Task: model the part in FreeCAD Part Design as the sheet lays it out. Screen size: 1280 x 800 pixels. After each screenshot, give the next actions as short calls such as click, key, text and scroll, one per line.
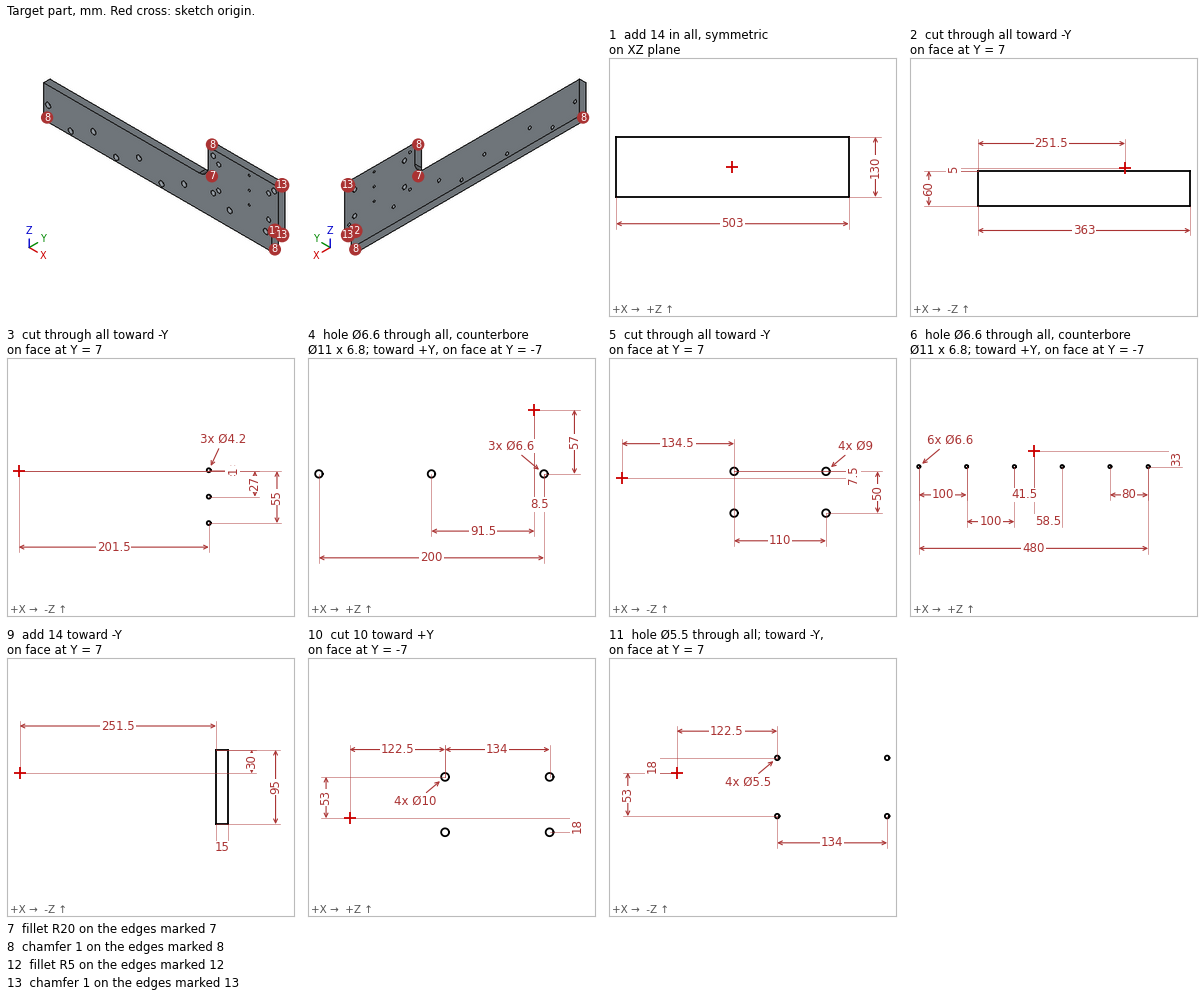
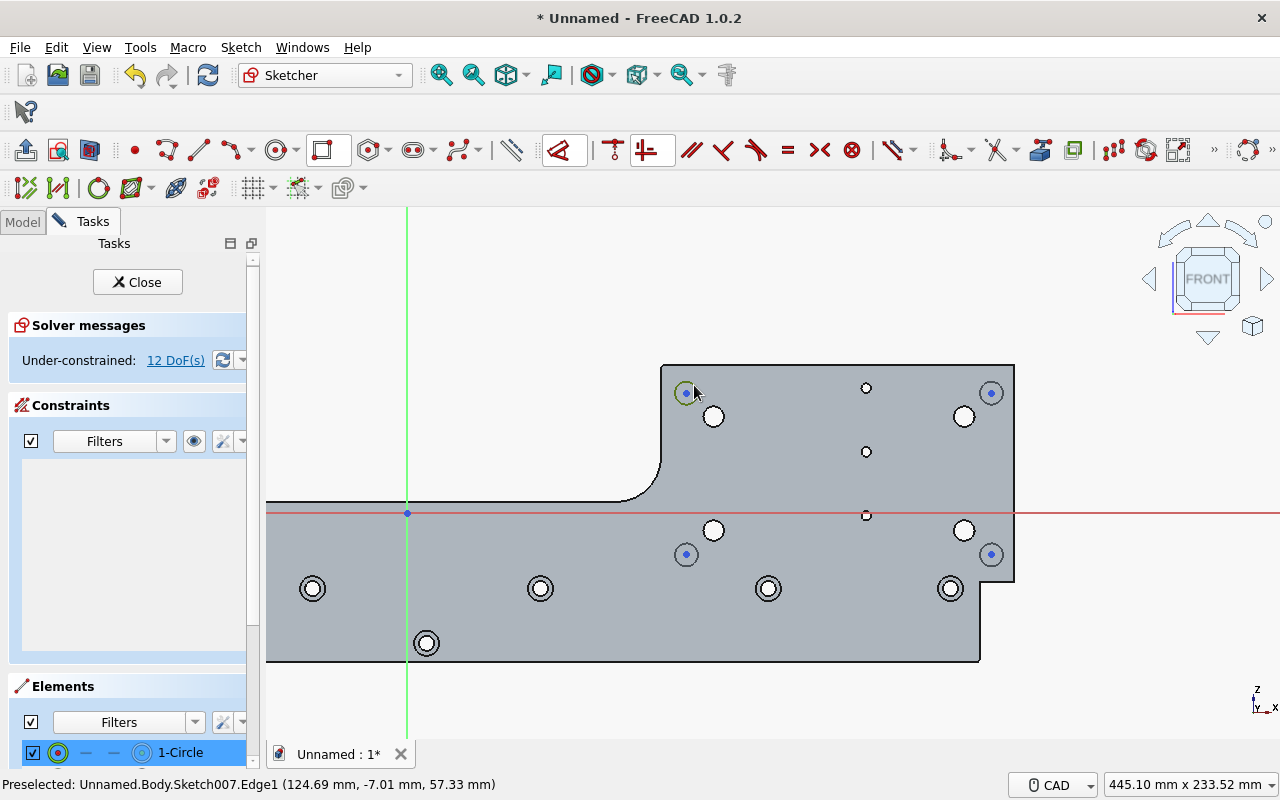
click(1000, 385)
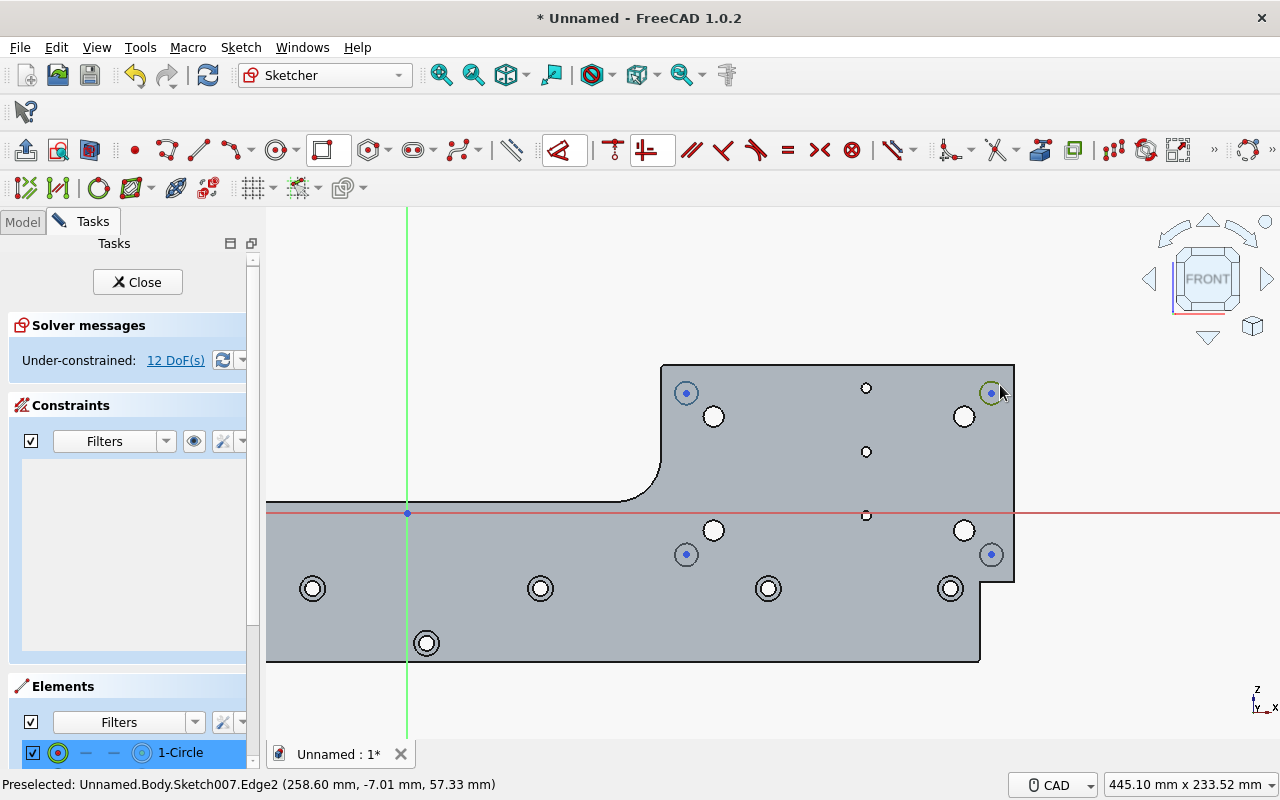
click(1000, 547)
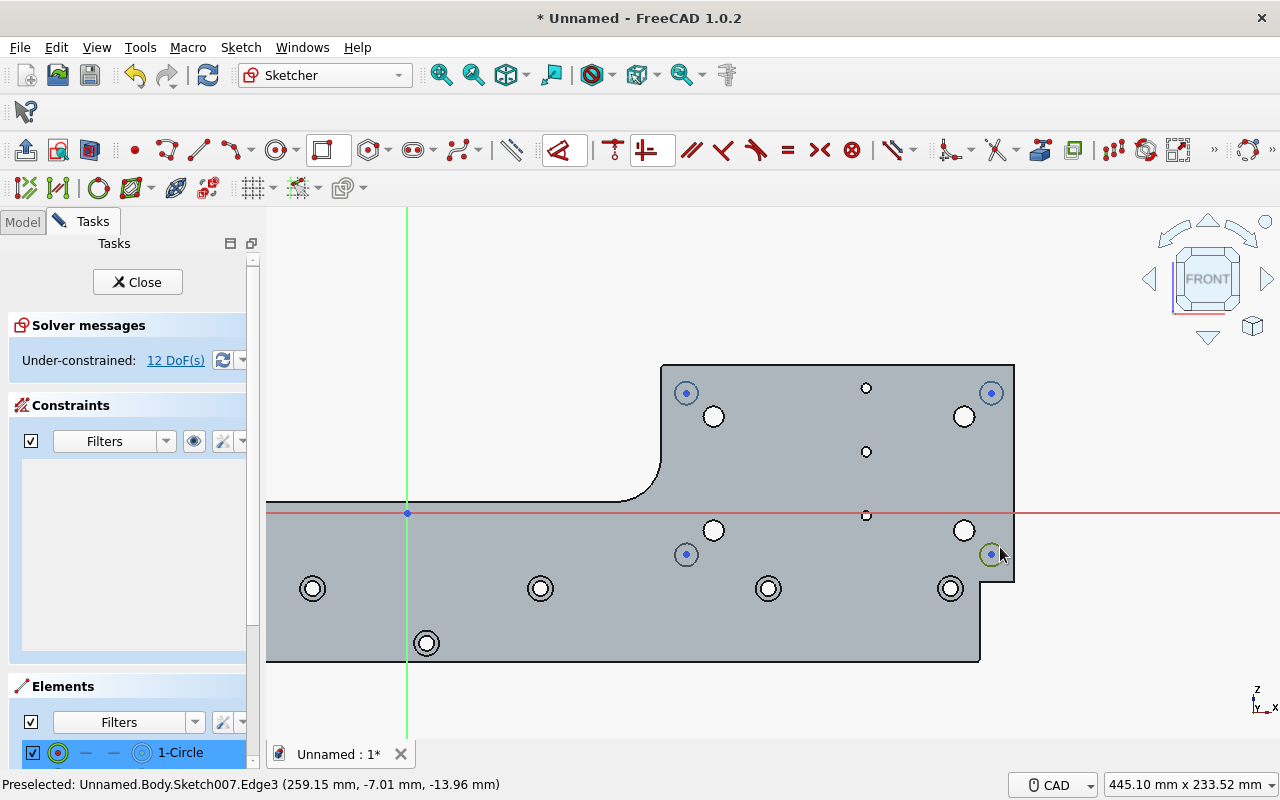
click(694, 547)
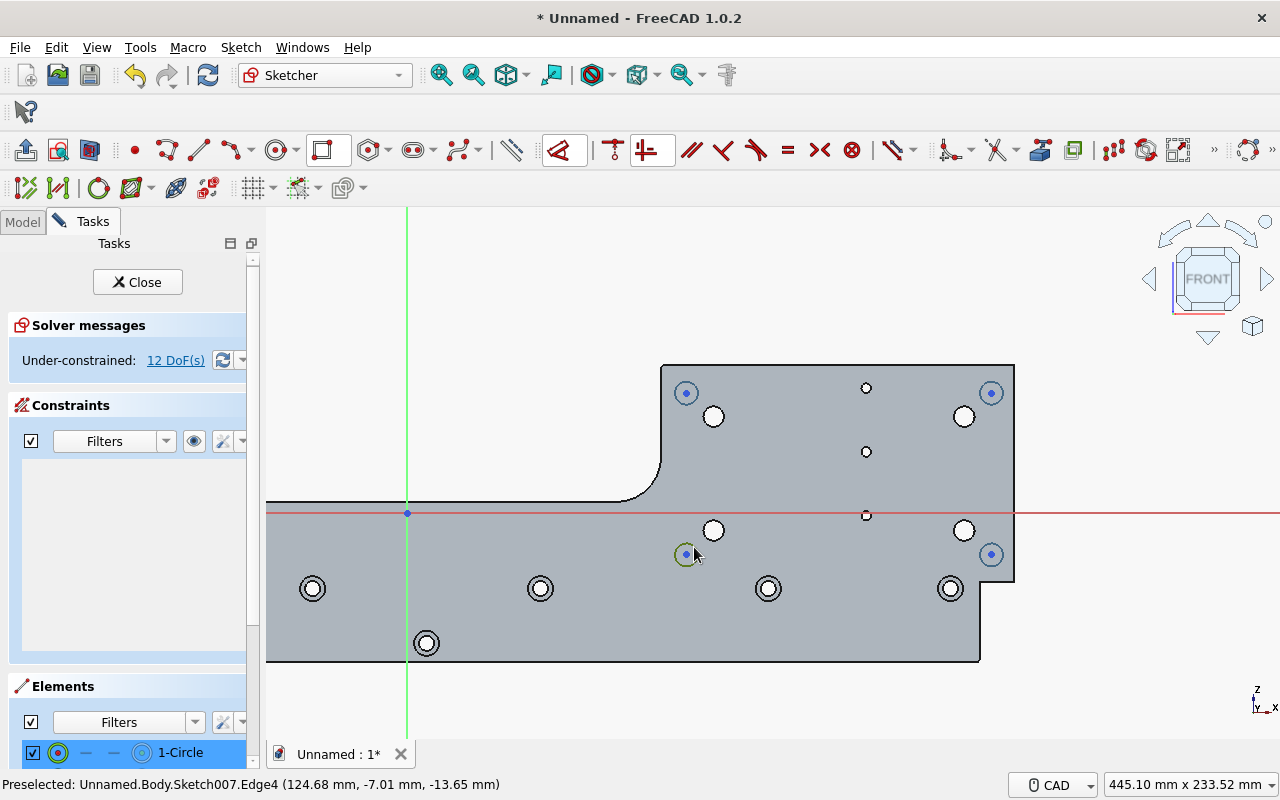
click(788, 150)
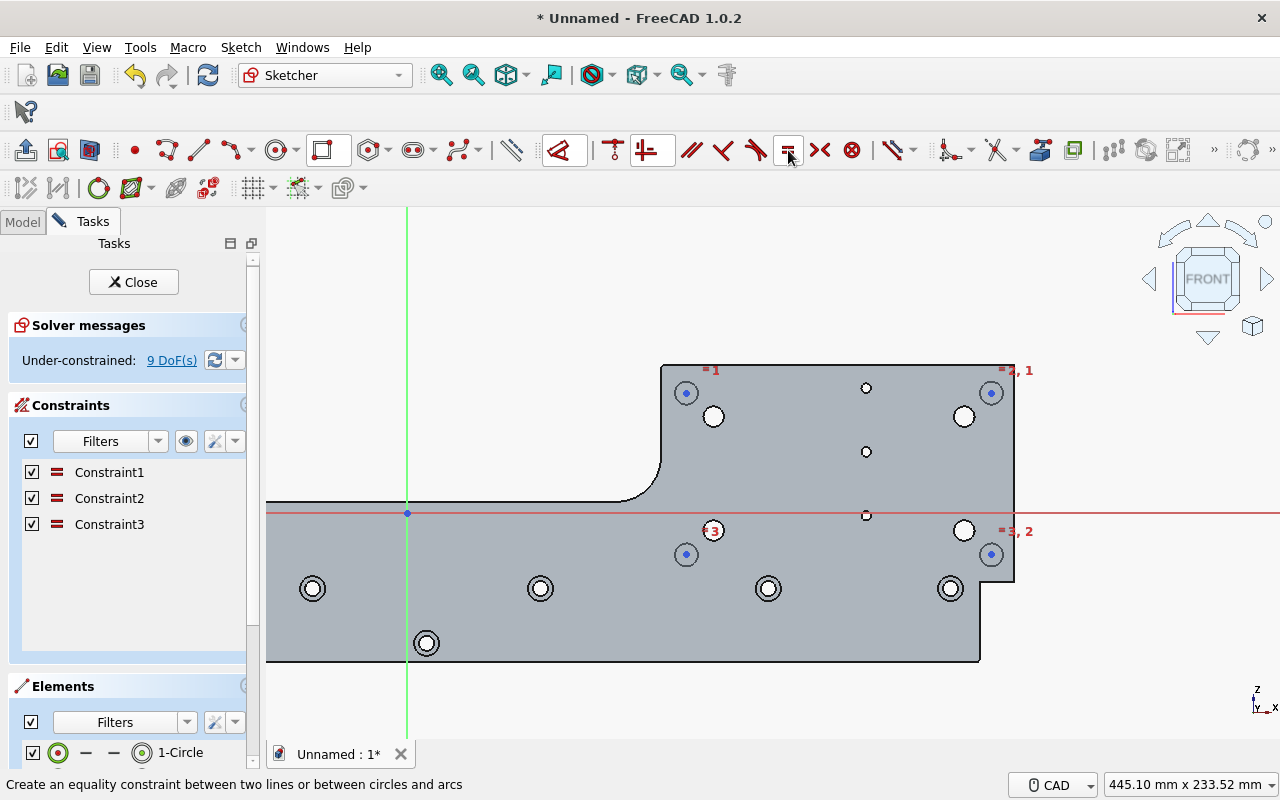
click(686, 393)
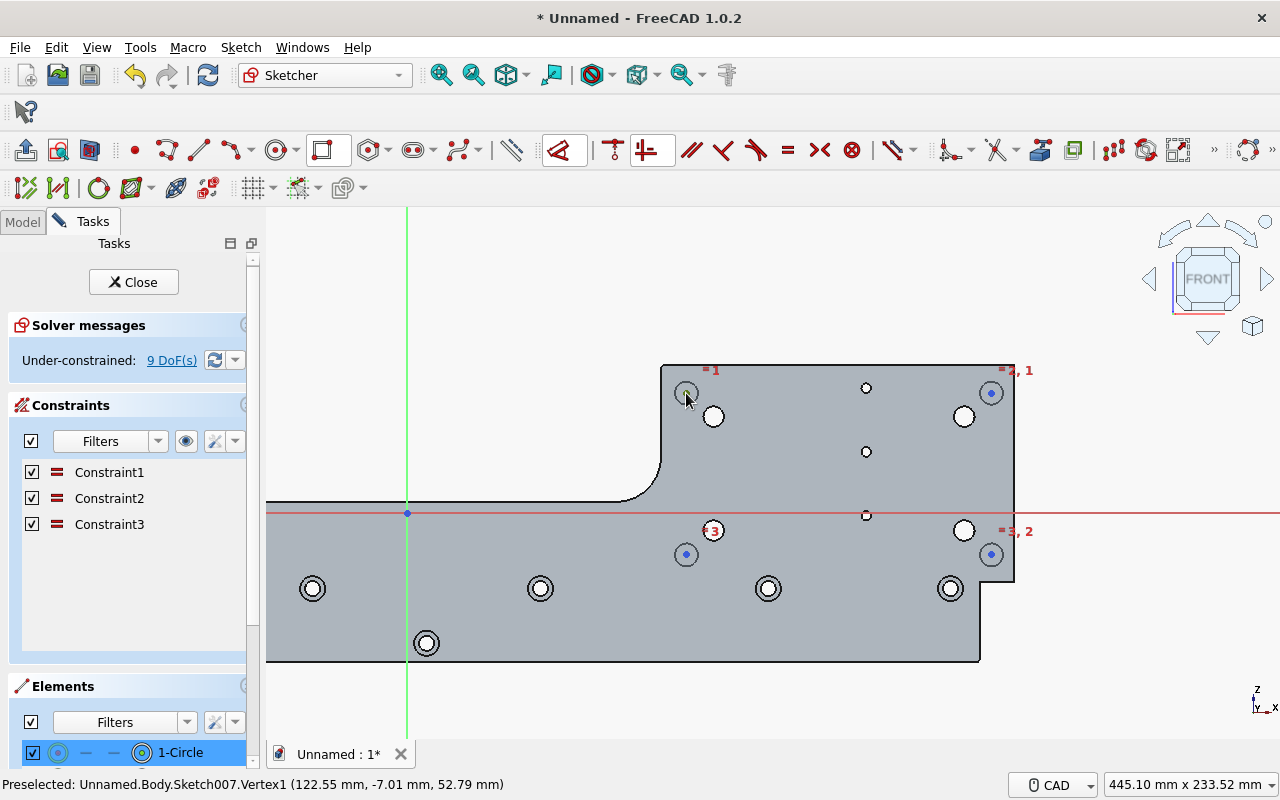
click(991, 393)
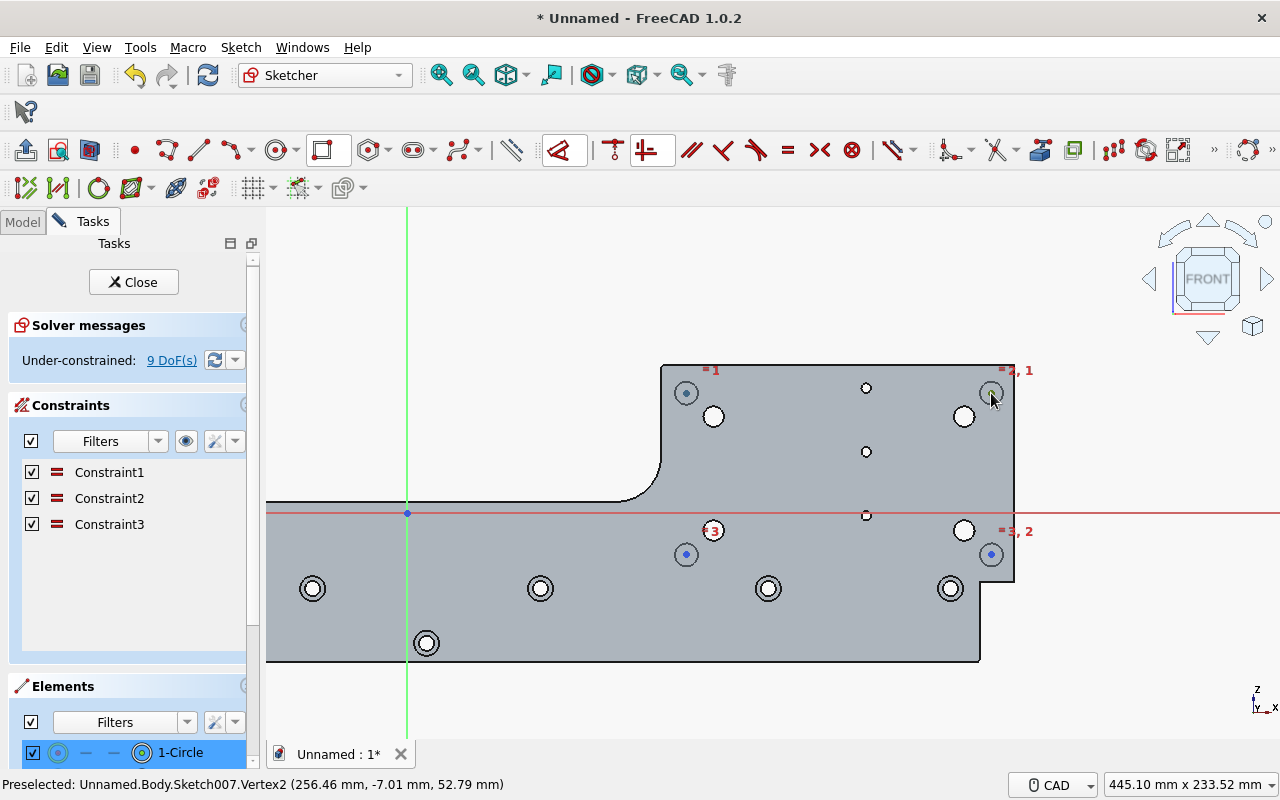
key(h)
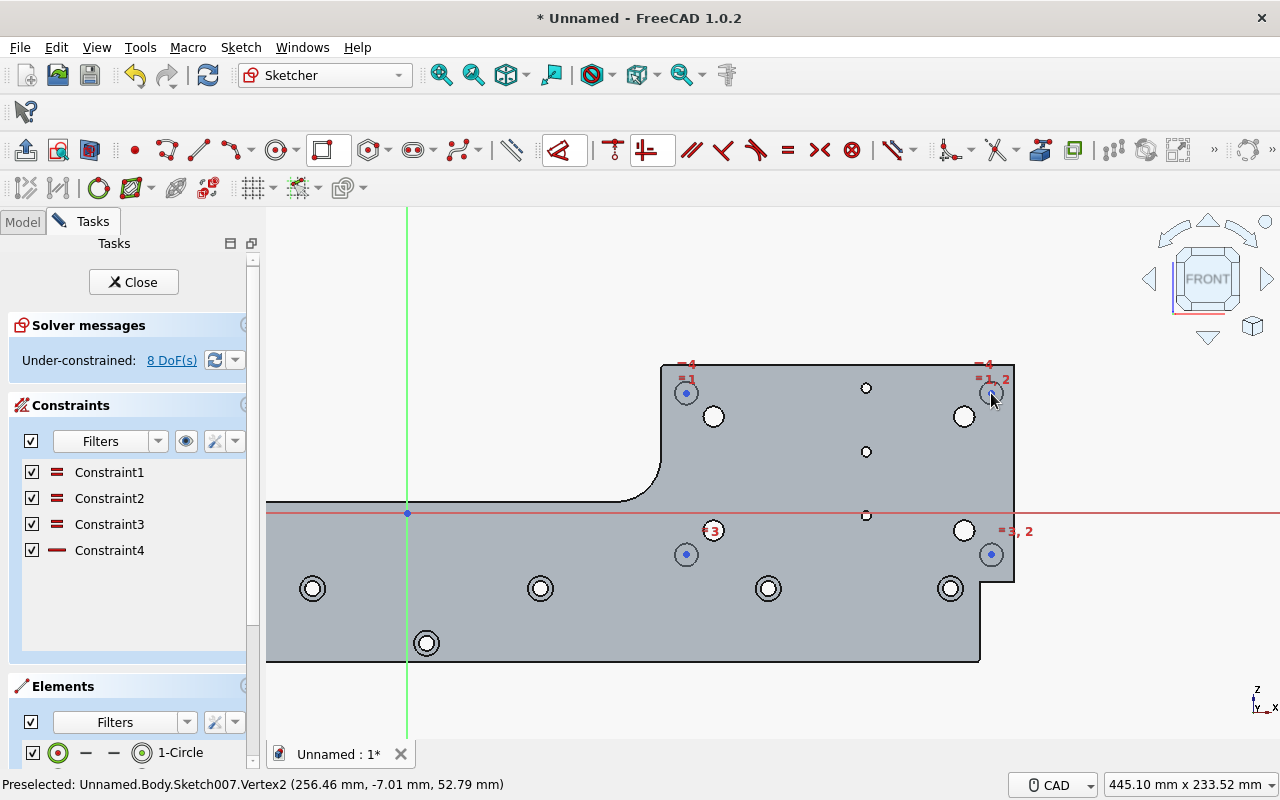
click(991, 393)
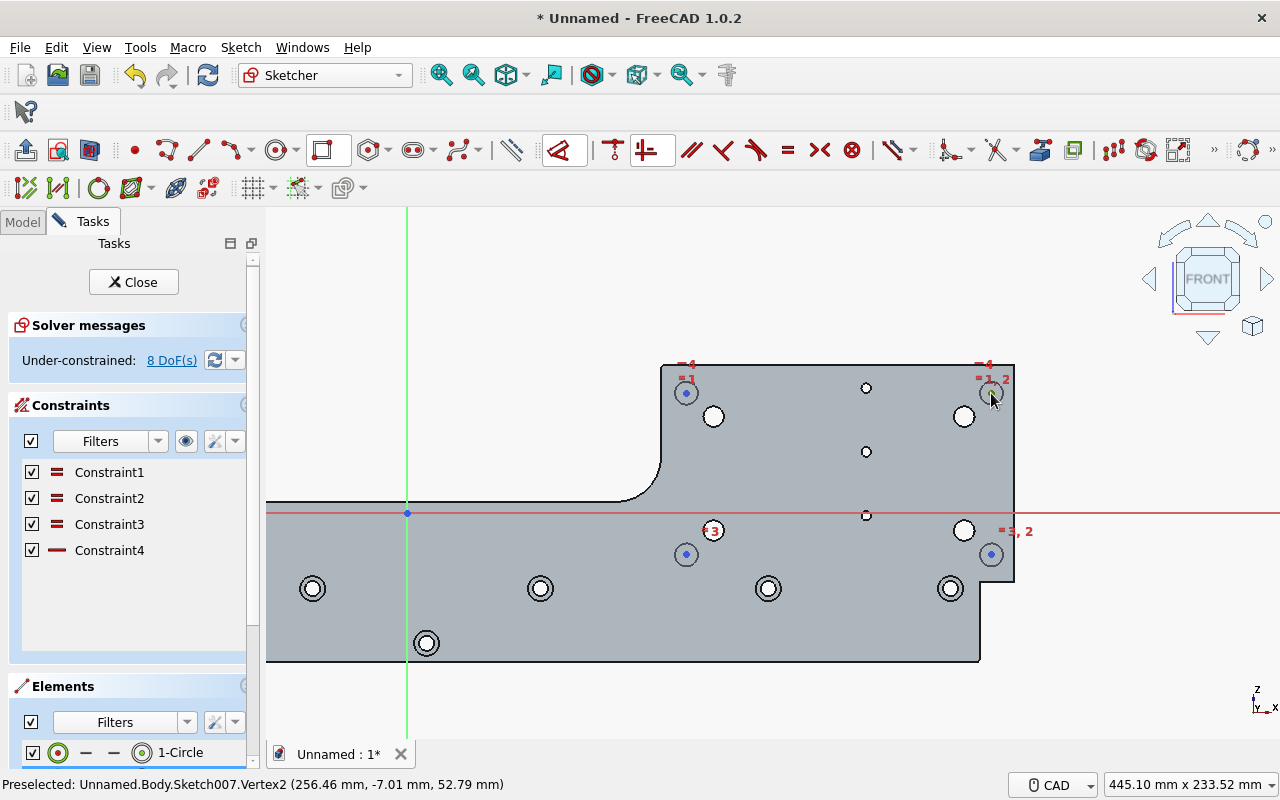
click(991, 555)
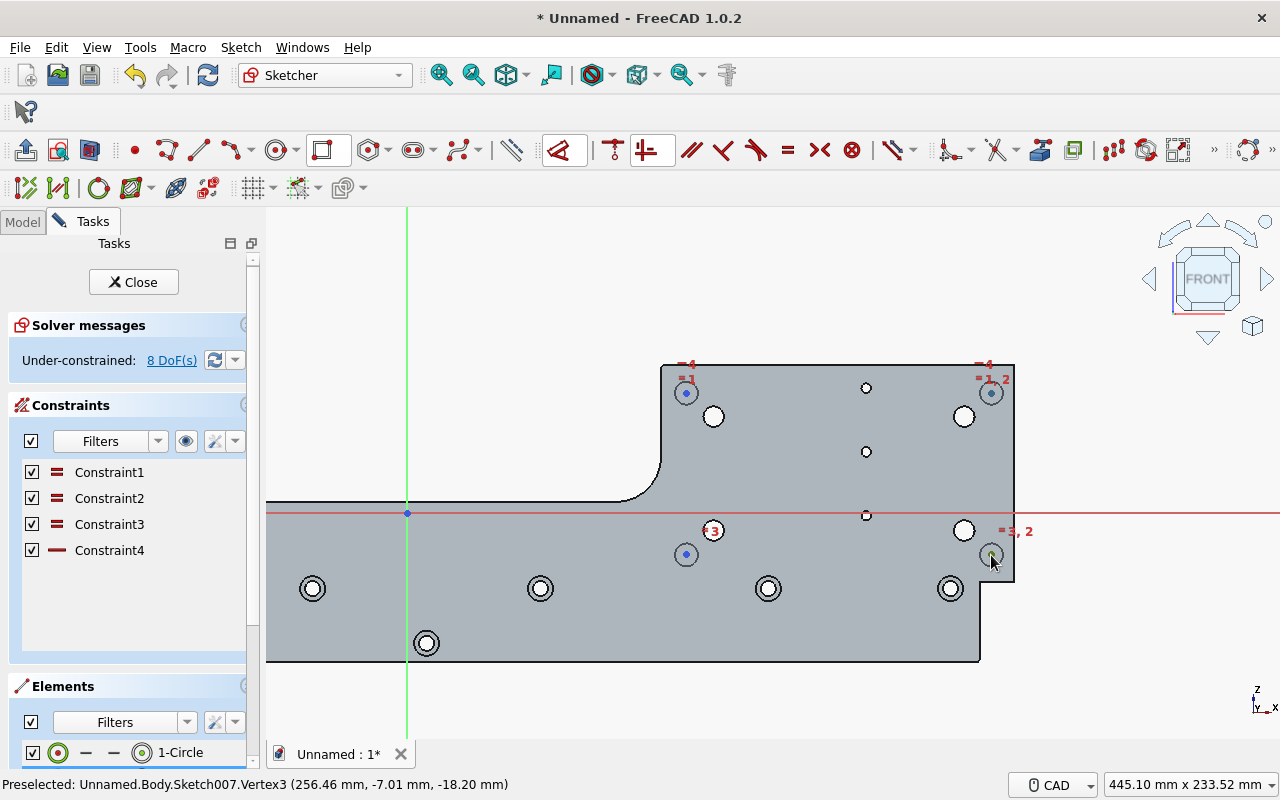
key(v)